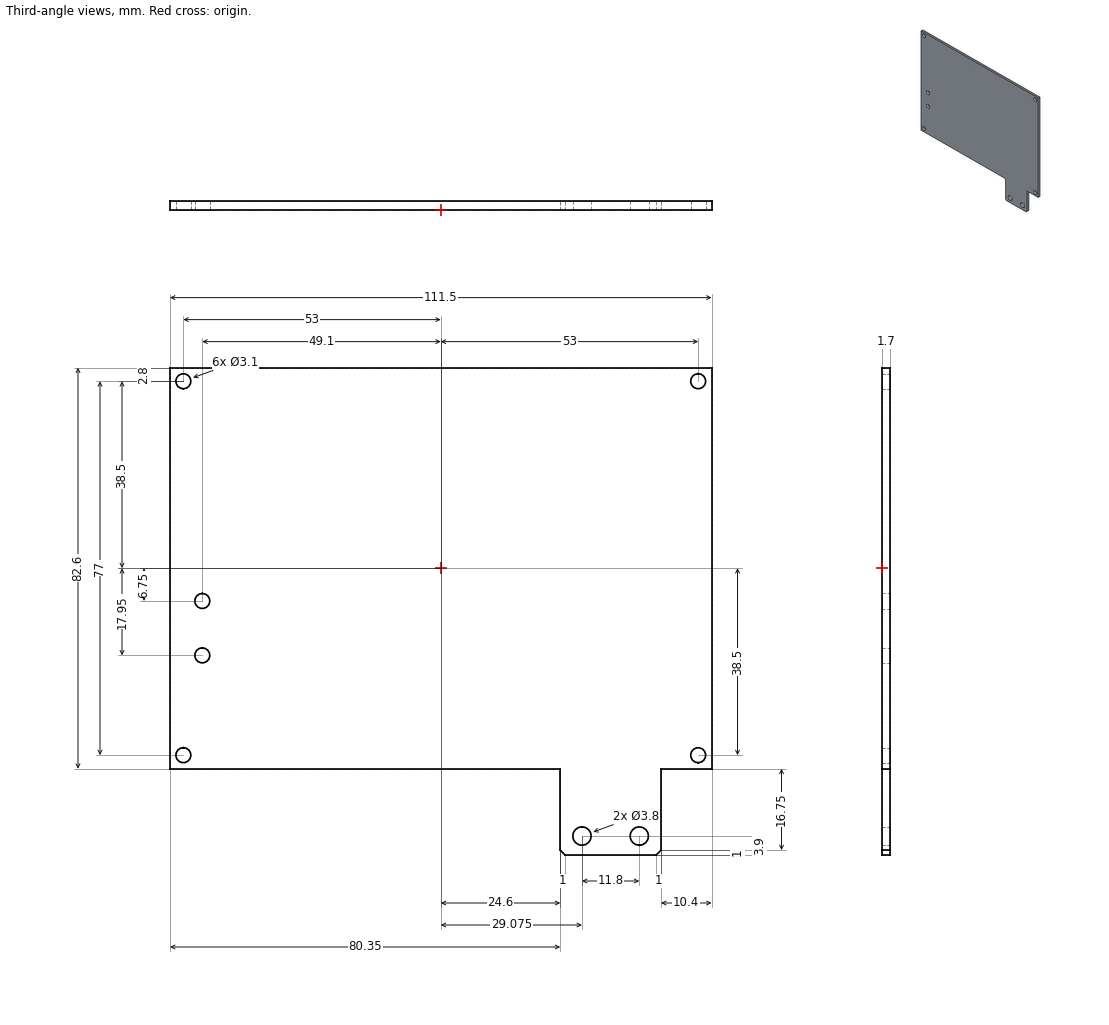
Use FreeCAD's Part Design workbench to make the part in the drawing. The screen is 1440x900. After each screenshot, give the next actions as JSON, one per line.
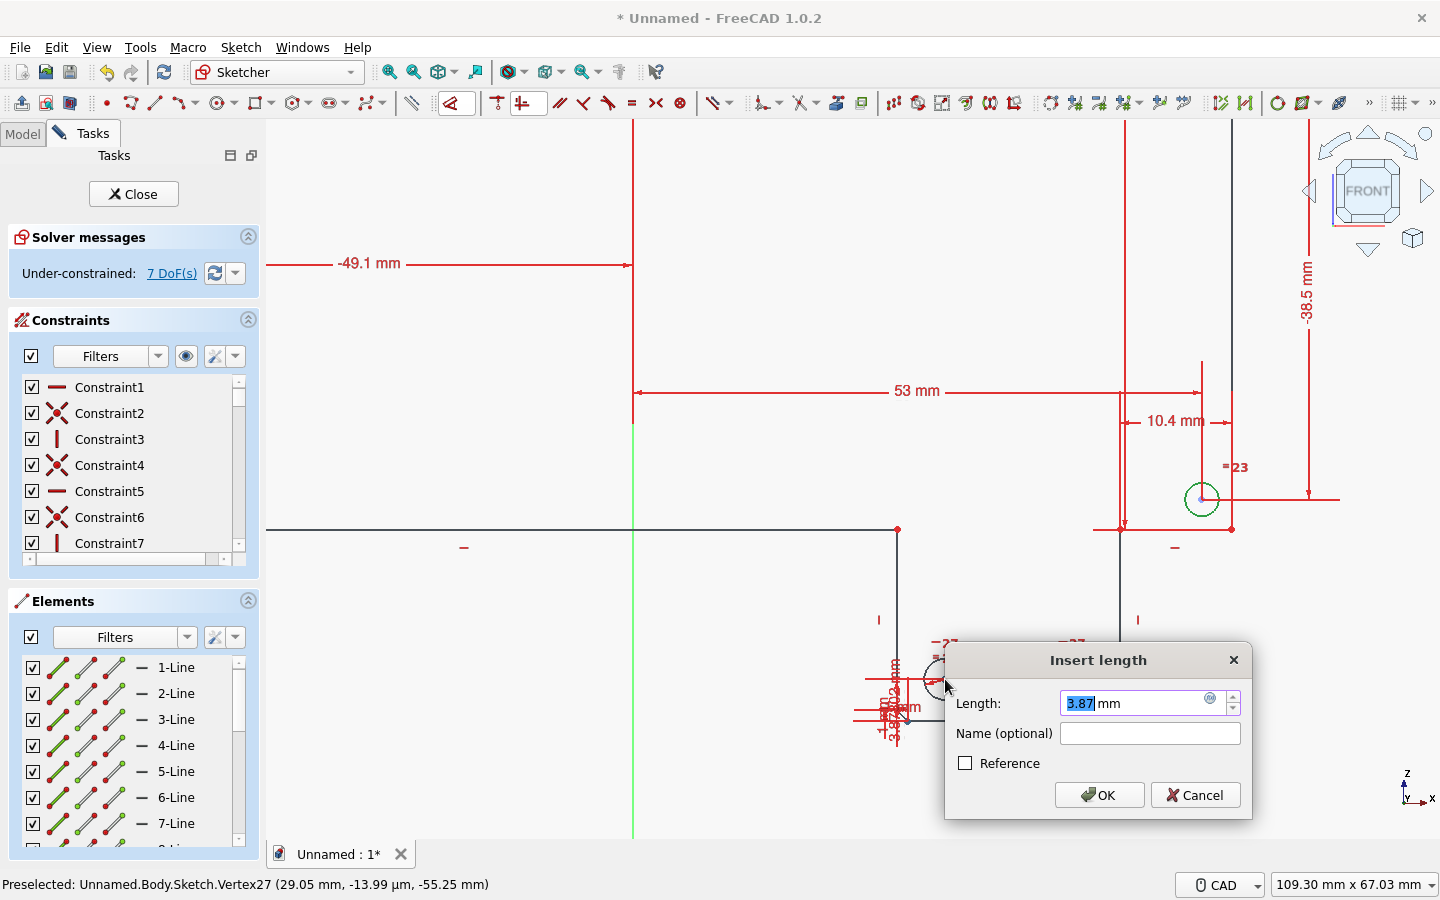
{"action": "type", "text": "3.9"}
{"action": "key", "text": "Return"}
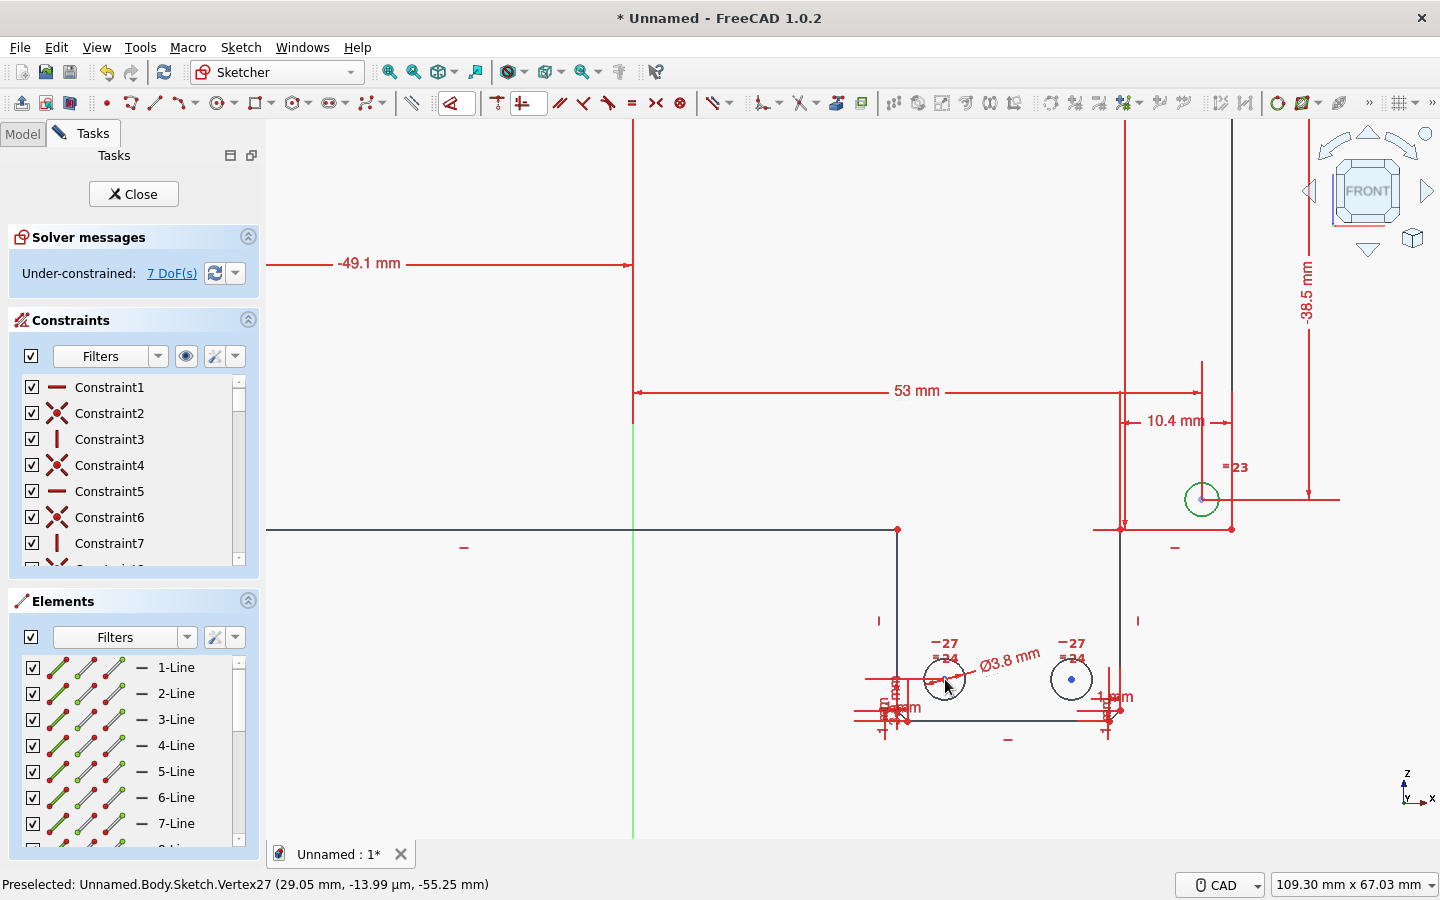
{"action": "left_click", "coordinate": [551, 530]}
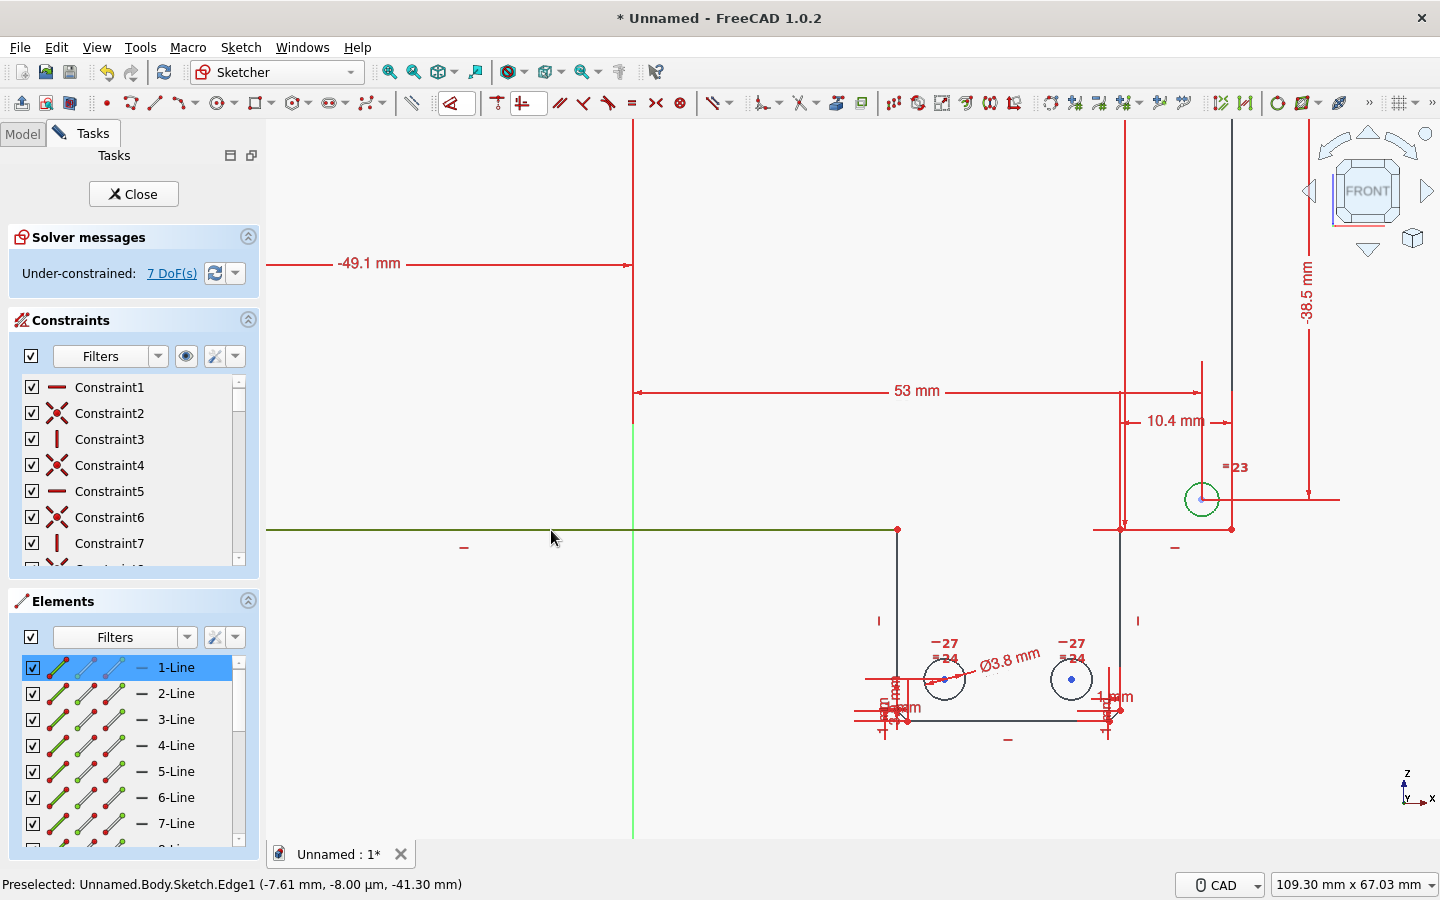
{"action": "left_click", "coordinate": [470, 104]}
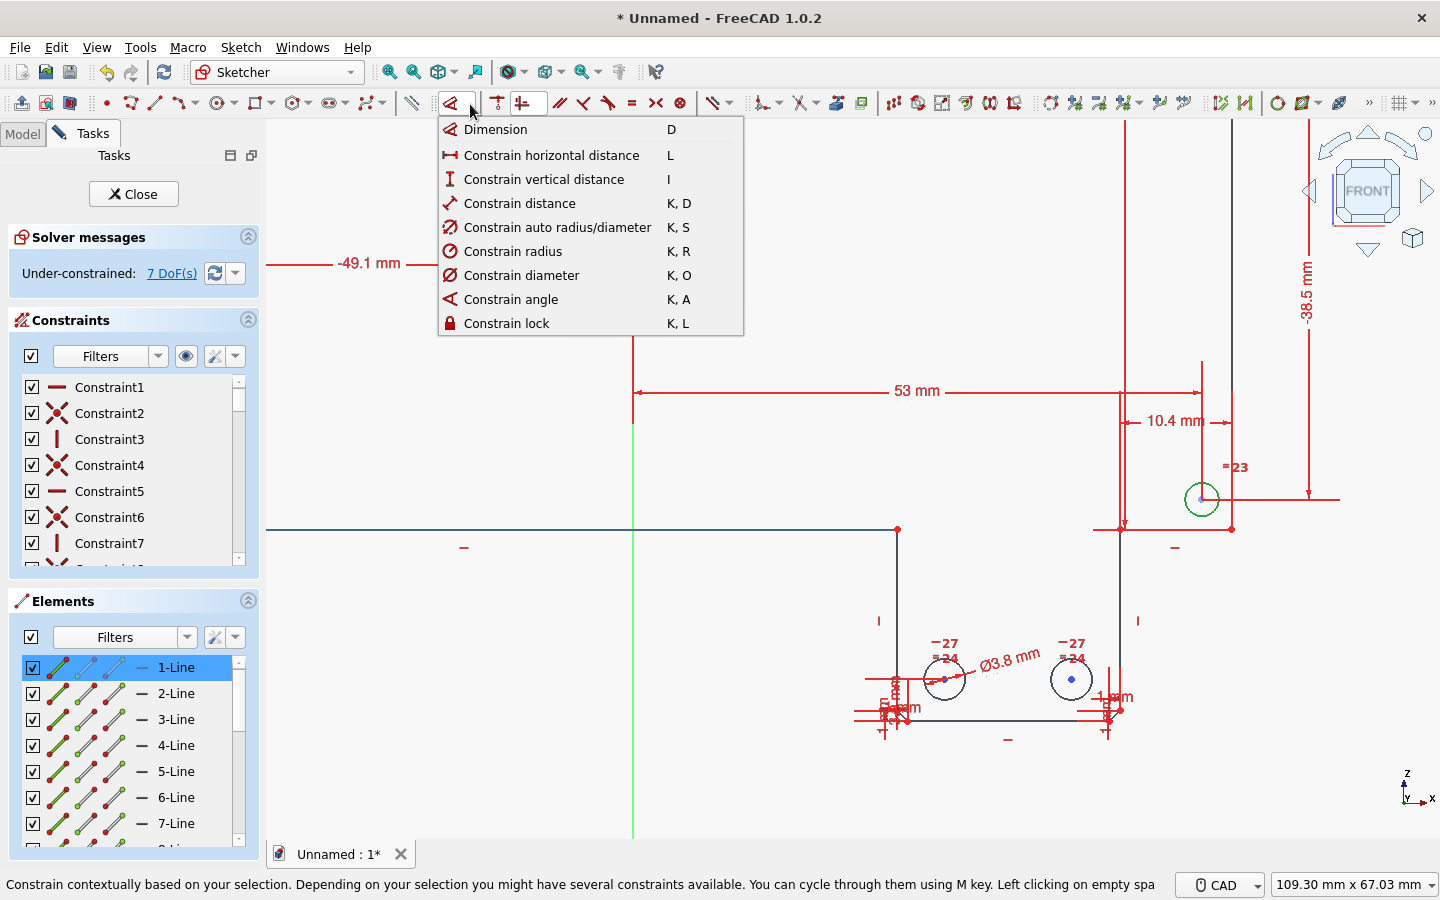
{"action": "left_click", "coordinate": [591, 155]}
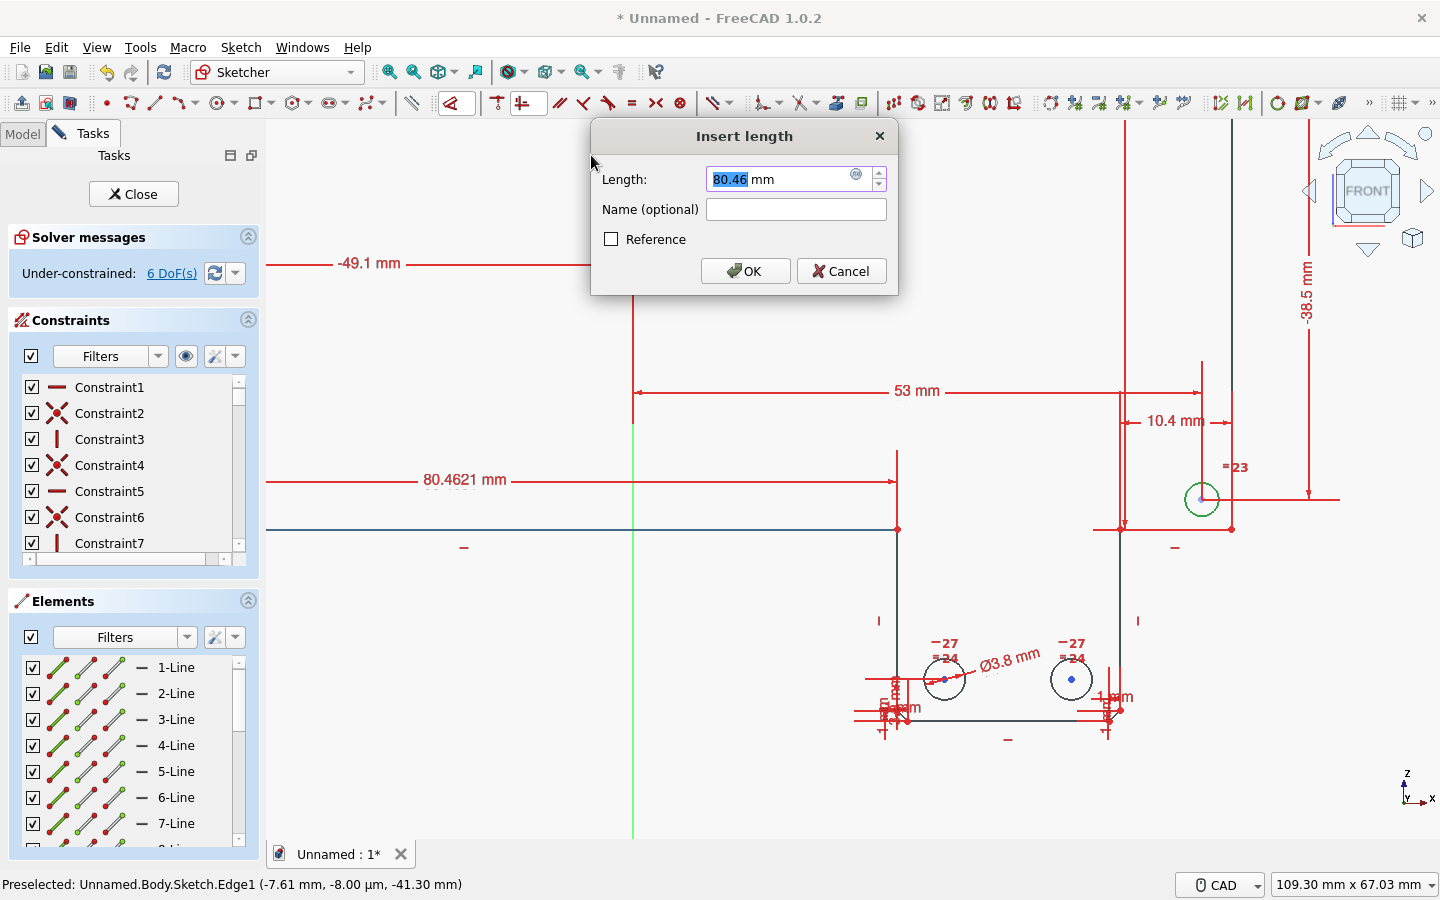
{"action": "type", "text": "80.35"}
{"action": "key", "text": "Return"}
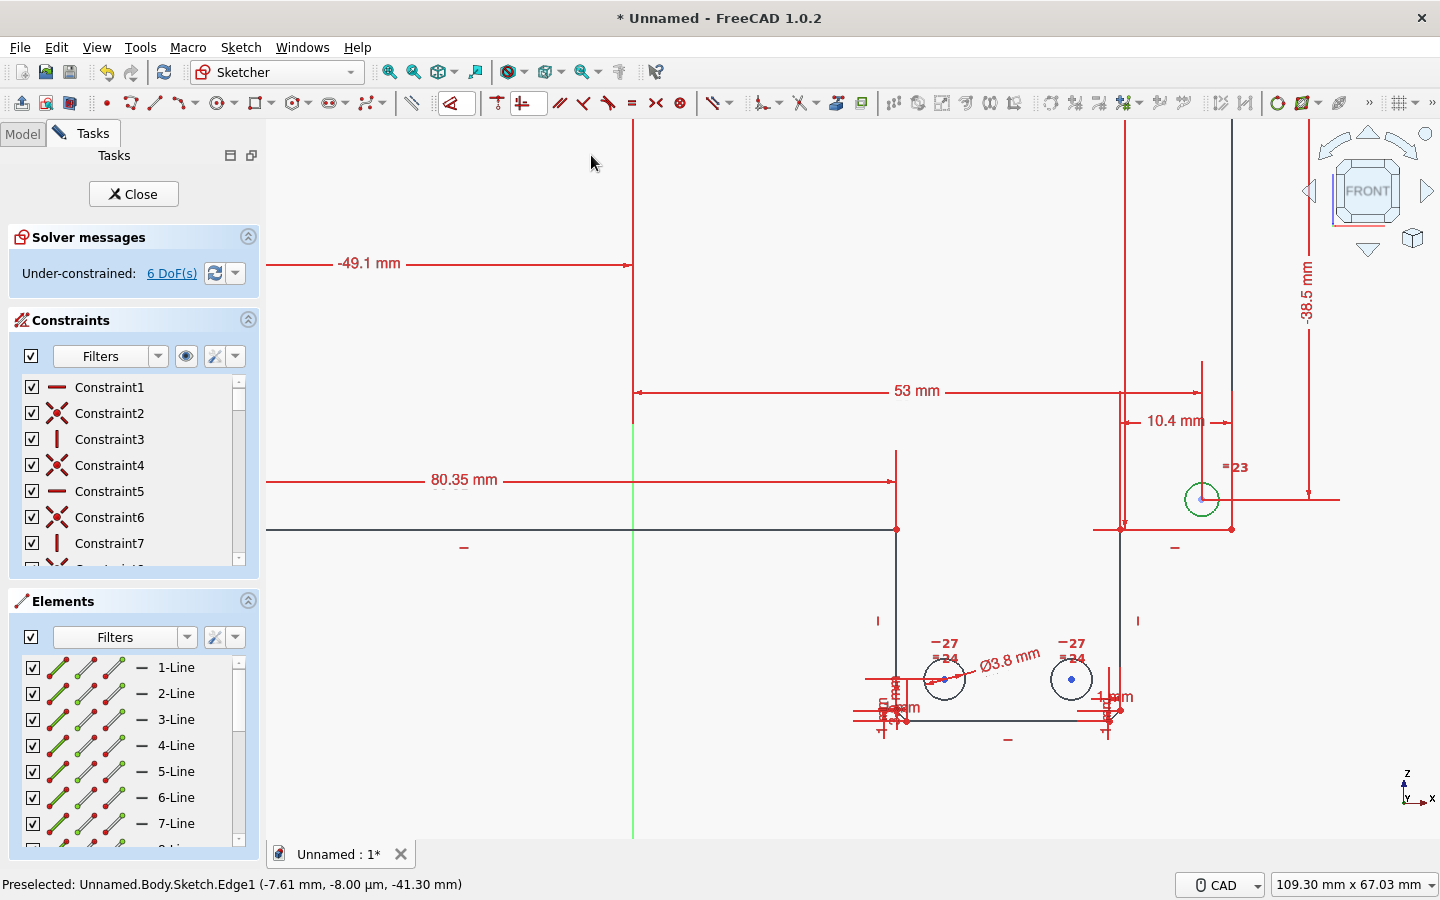
{"action": "scroll", "coordinate": [908, 722], "scroll_direction": "down", "scroll_amount": 4}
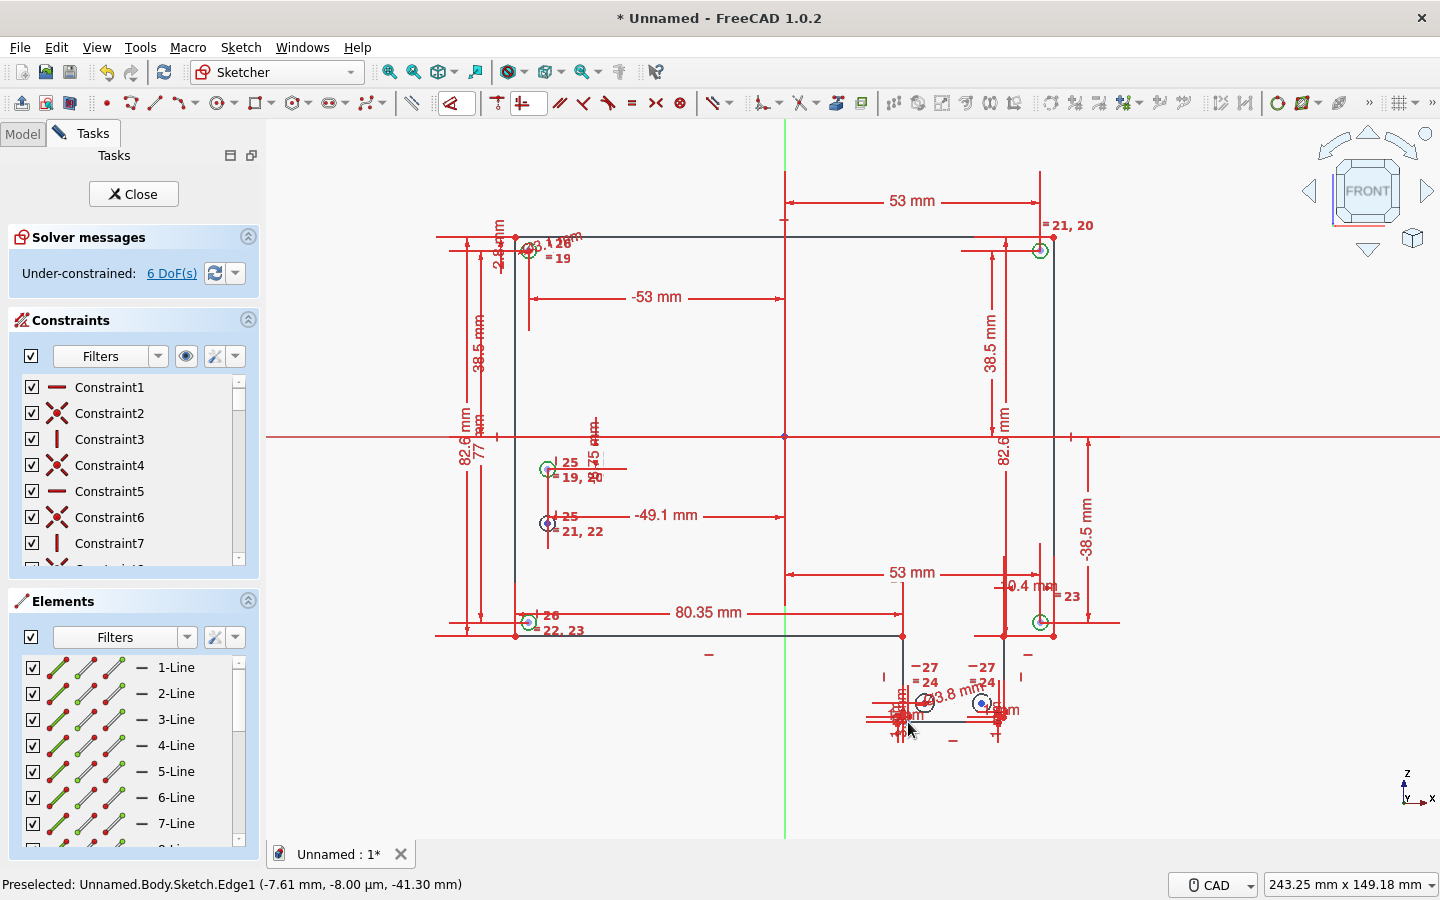
{"action": "left_click", "coordinate": [677, 237]}